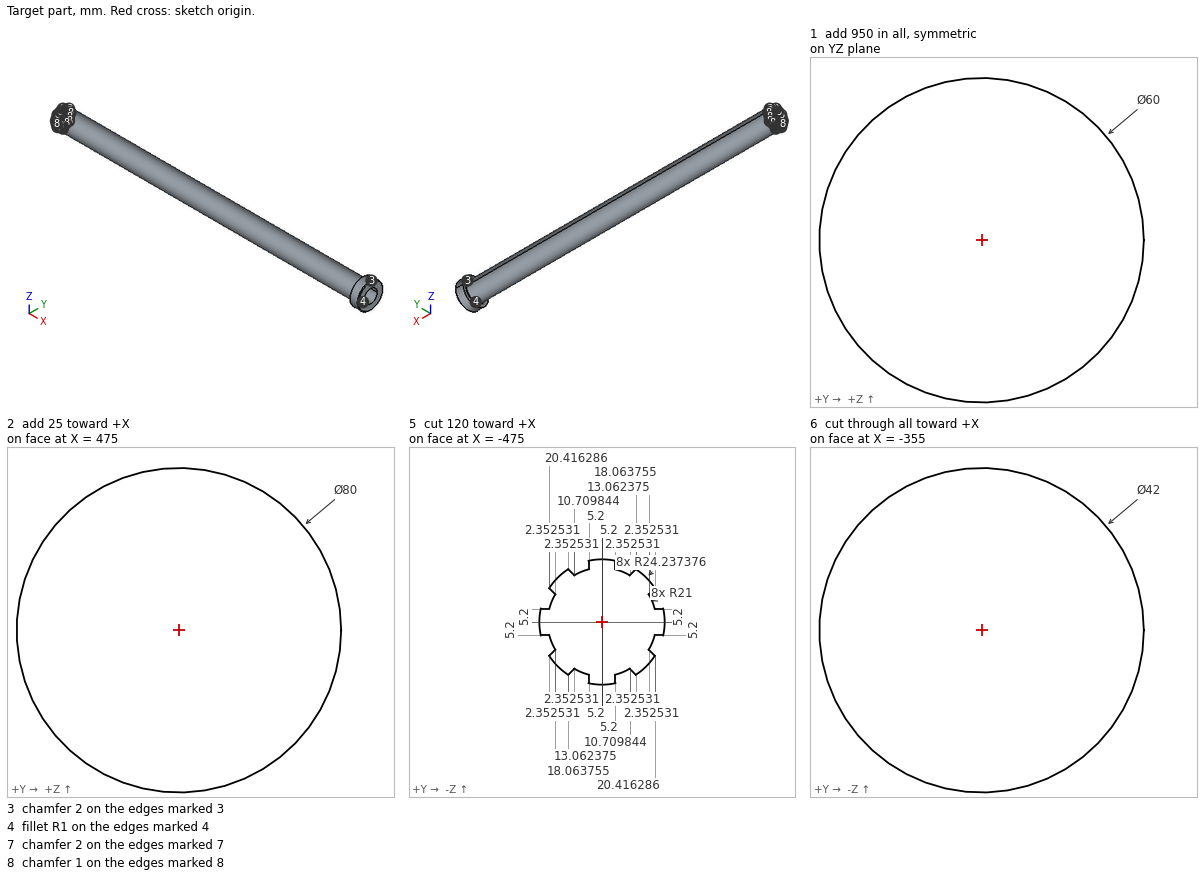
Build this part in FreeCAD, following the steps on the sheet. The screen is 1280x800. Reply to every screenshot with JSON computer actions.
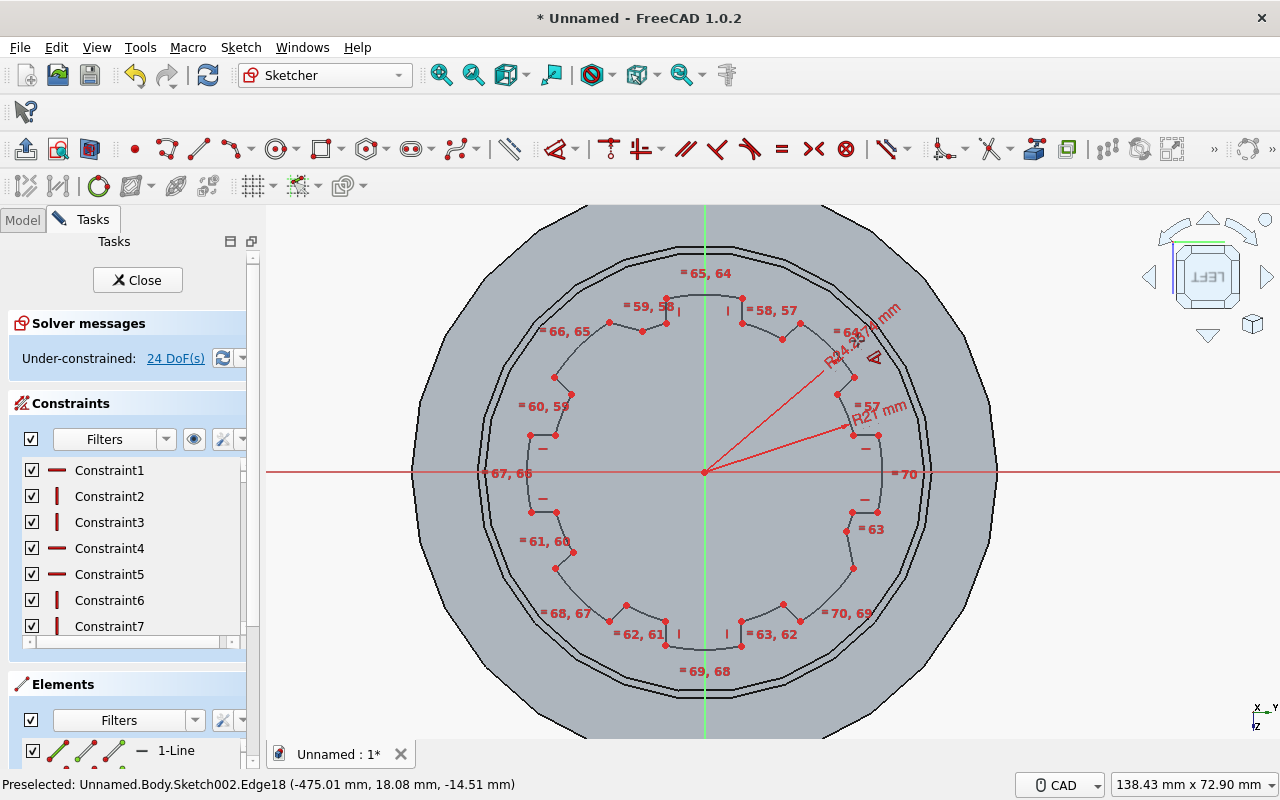
{"action": "left_click", "coordinate": [878, 435]}
{"action": "left_click", "coordinate": [912, 454]}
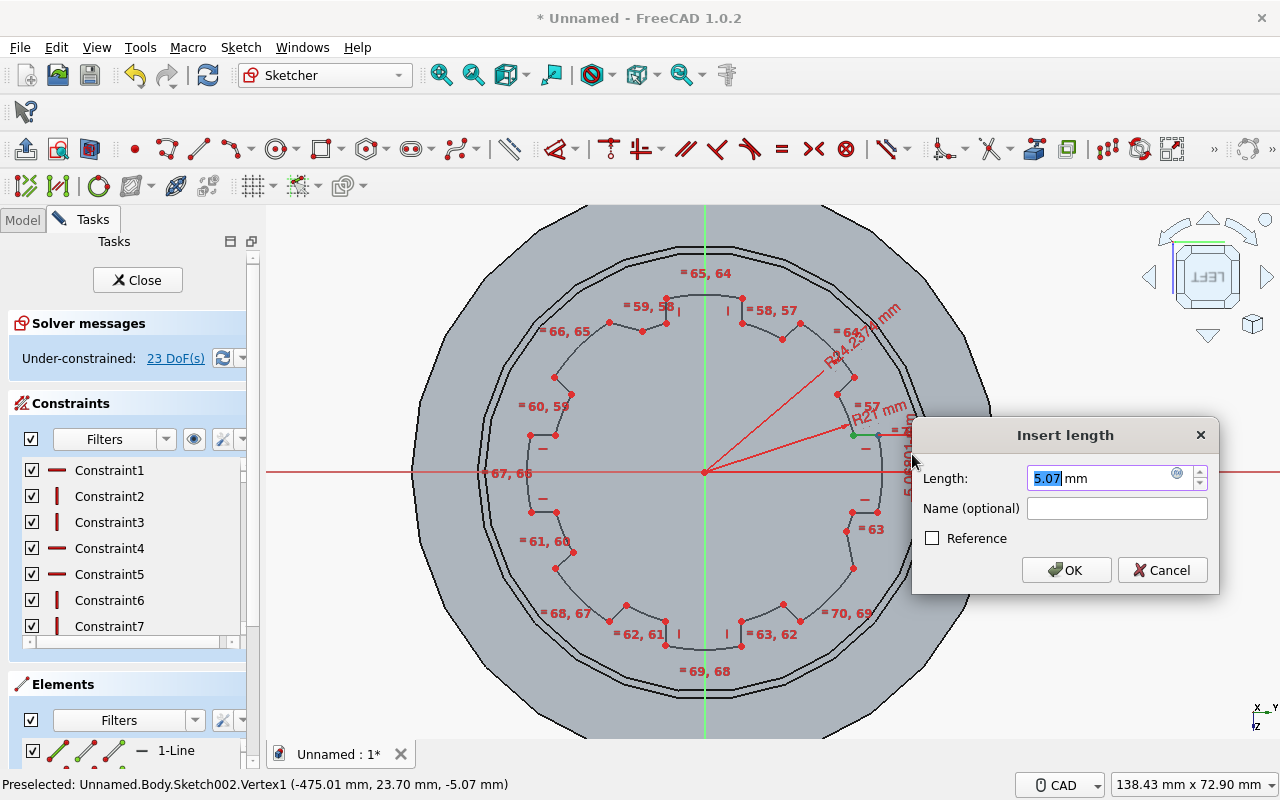
{"action": "type", "text": "5.2"}
{"action": "key", "text": "Return"}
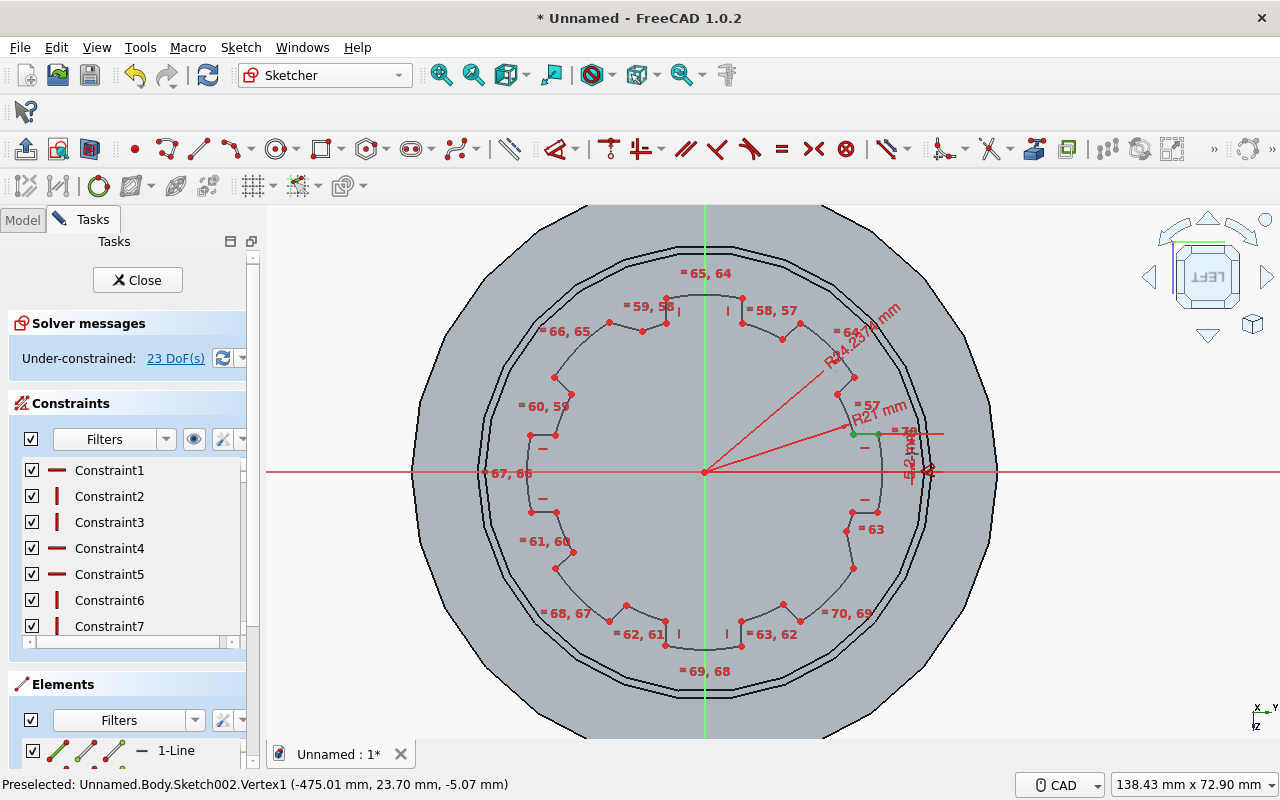
{"action": "left_click", "coordinate": [742, 323]}
{"action": "left_click", "coordinate": [723, 506]}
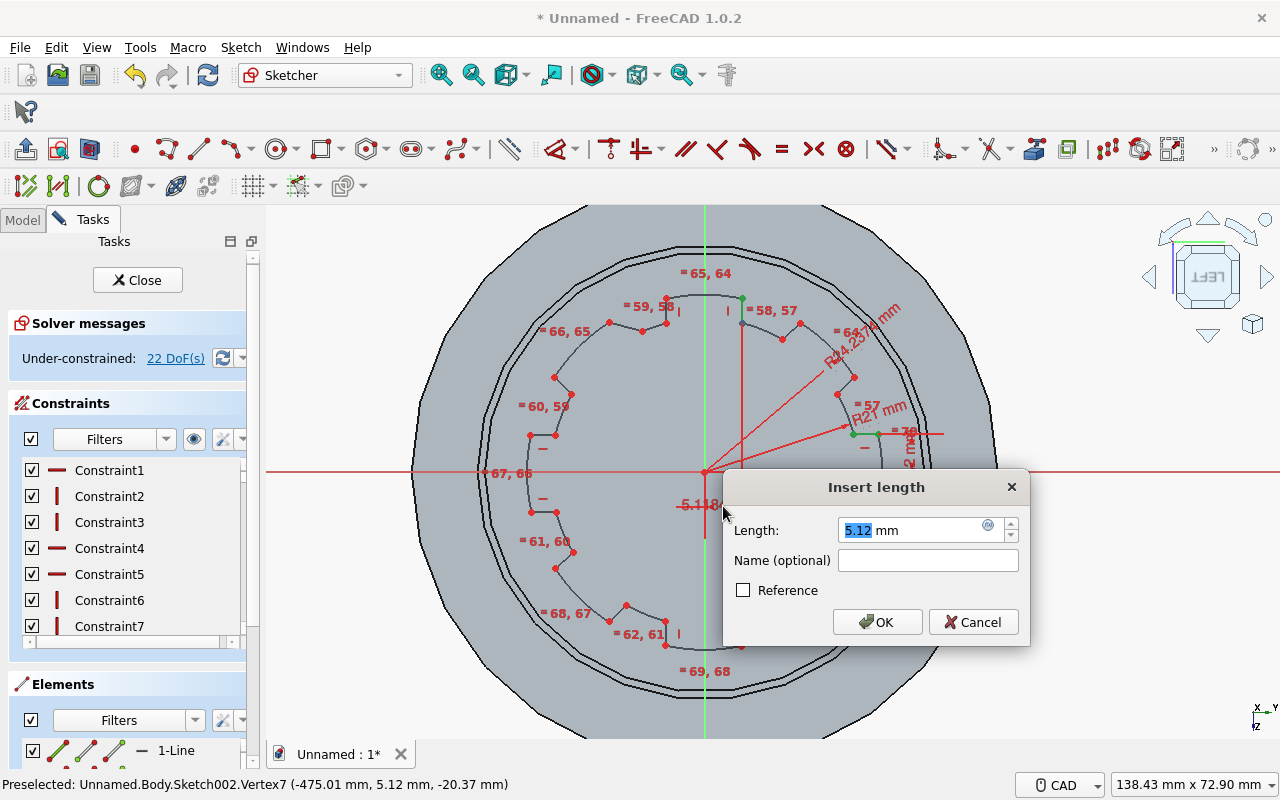
{"action": "type", "text": "5.2"}
{"action": "key", "text": "Return"}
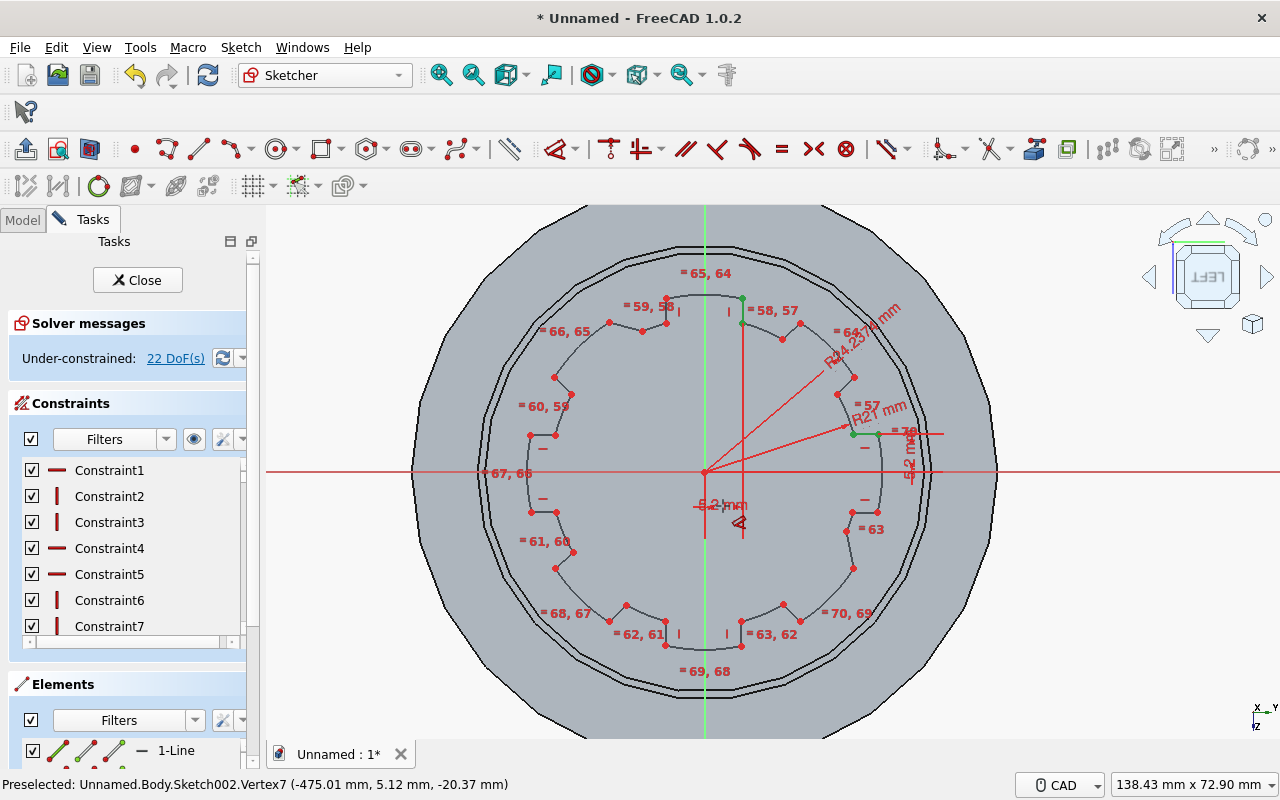
{"action": "left_click", "coordinate": [666, 299]}
{"action": "left_click", "coordinate": [686, 265]}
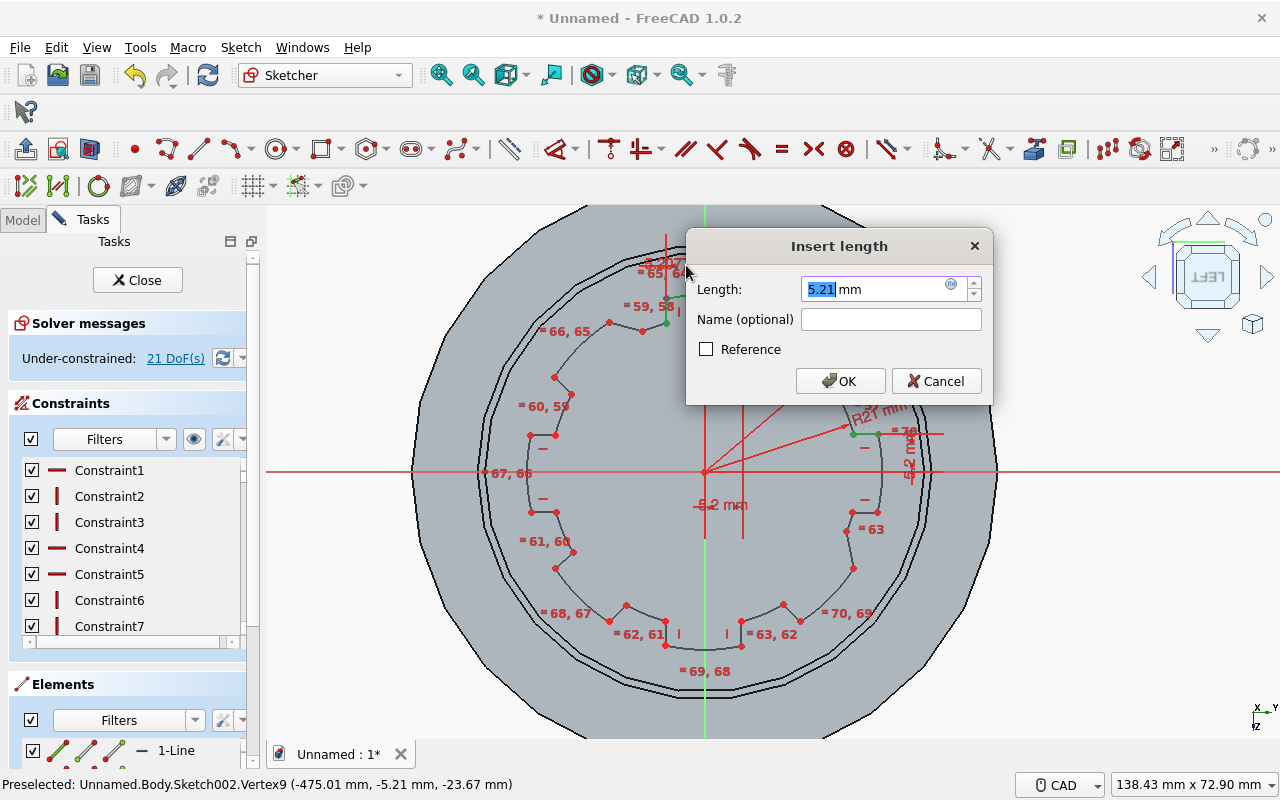
{"action": "type", "text": "5.2"}
{"action": "key", "text": "Return"}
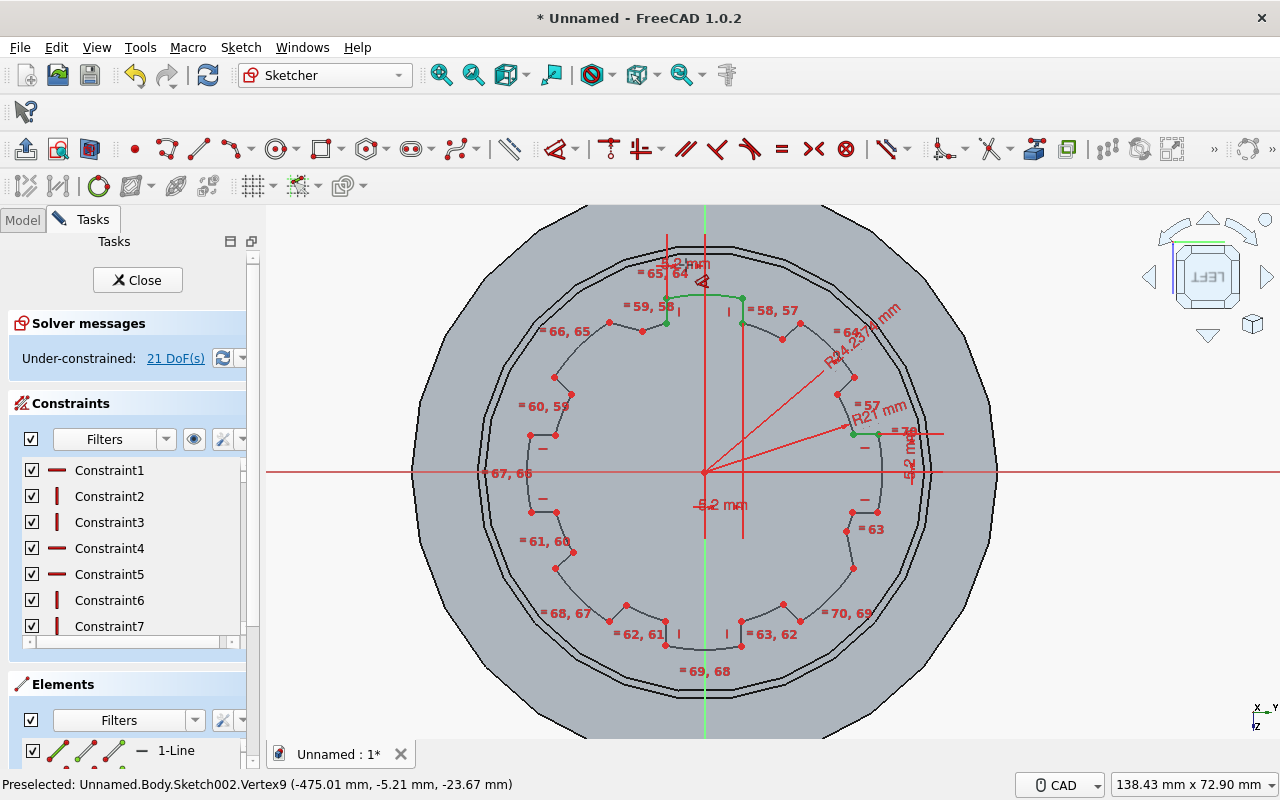
{"action": "left_click", "coordinate": [555, 435]}
{"action": "left_click", "coordinate": [739, 454]}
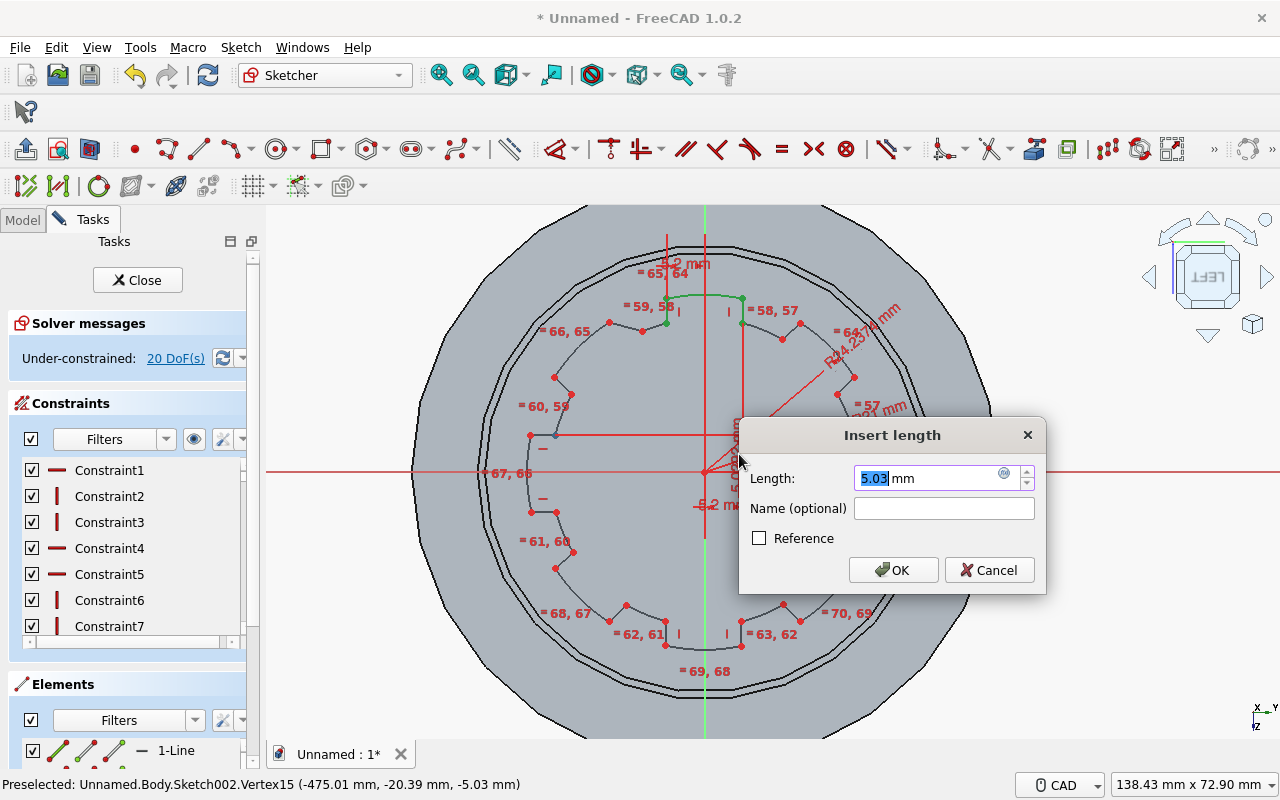
{"action": "type", "text": "5.2"}
{"action": "key", "text": "Return"}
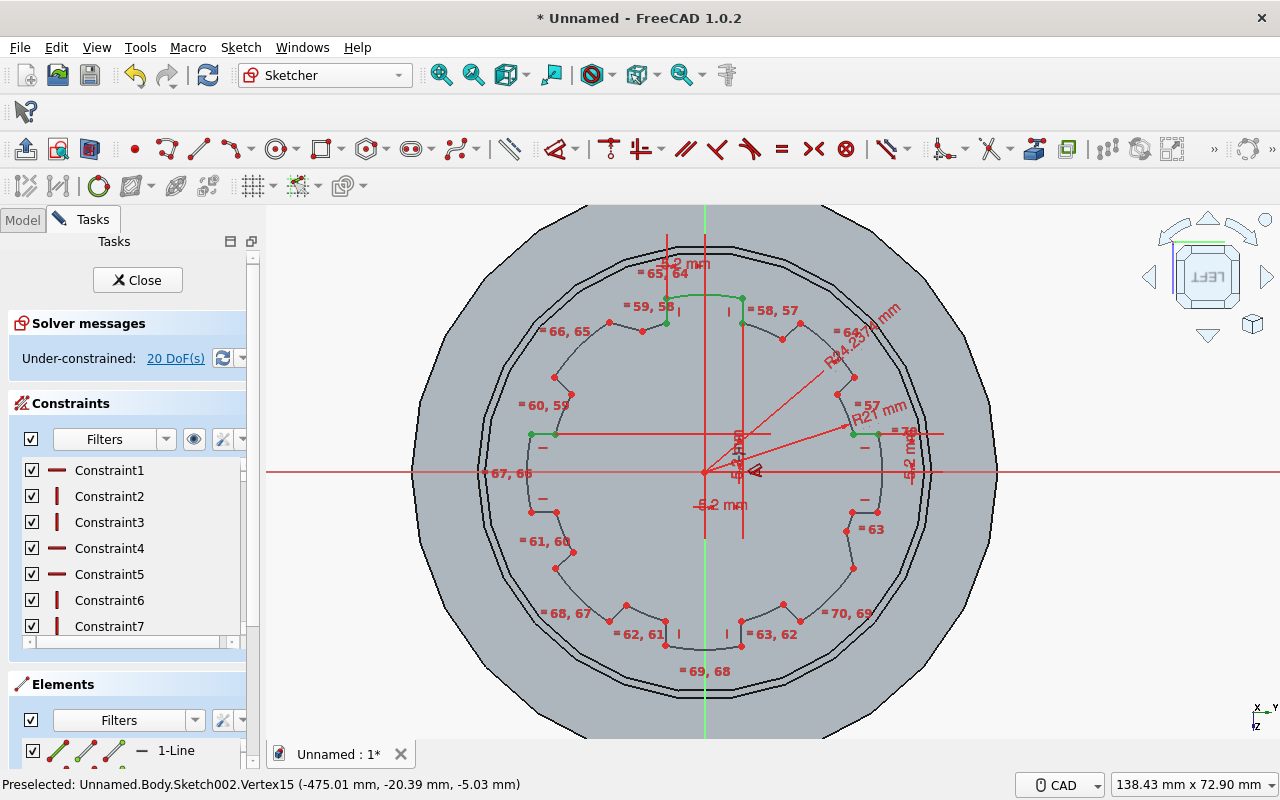
{"action": "left_click", "coordinate": [532, 512]}
{"action": "left_click", "coordinate": [498, 492]}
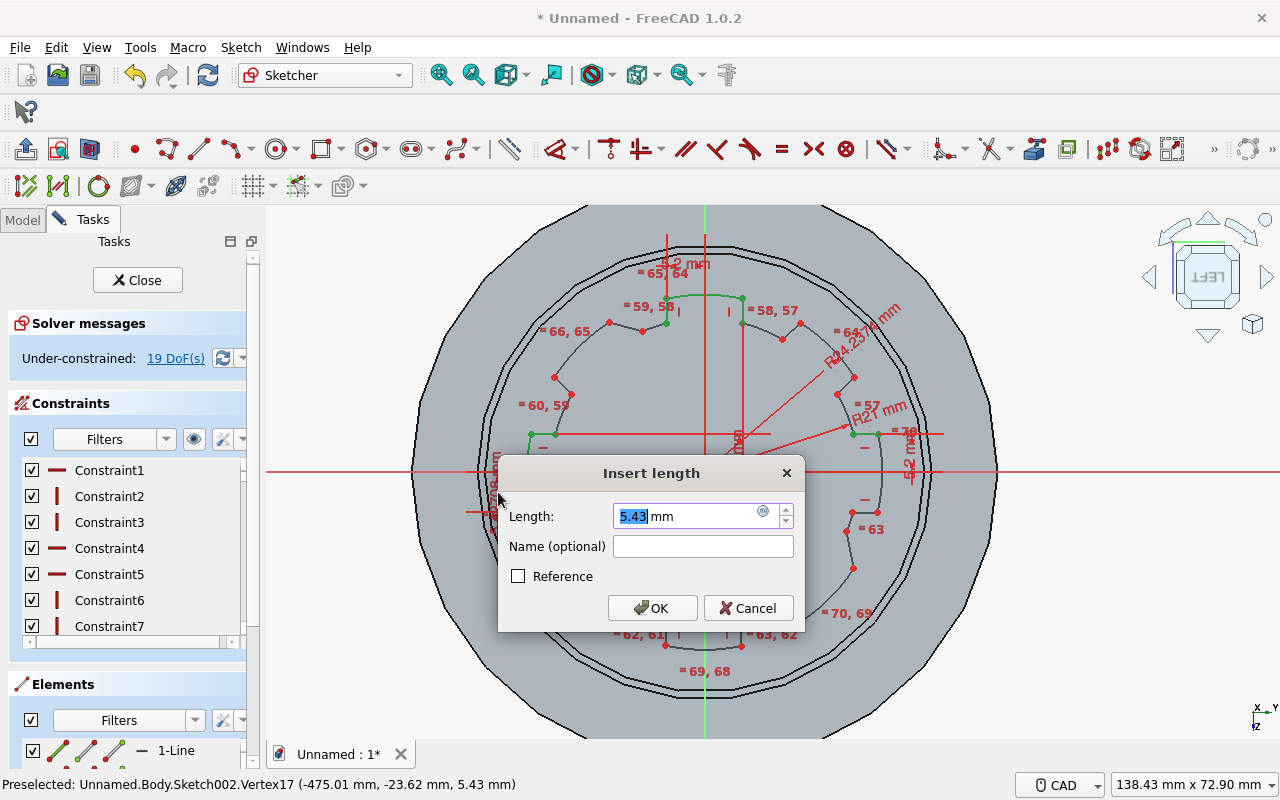
{"action": "type", "text": "5.2"}
{"action": "key", "text": "Return"}